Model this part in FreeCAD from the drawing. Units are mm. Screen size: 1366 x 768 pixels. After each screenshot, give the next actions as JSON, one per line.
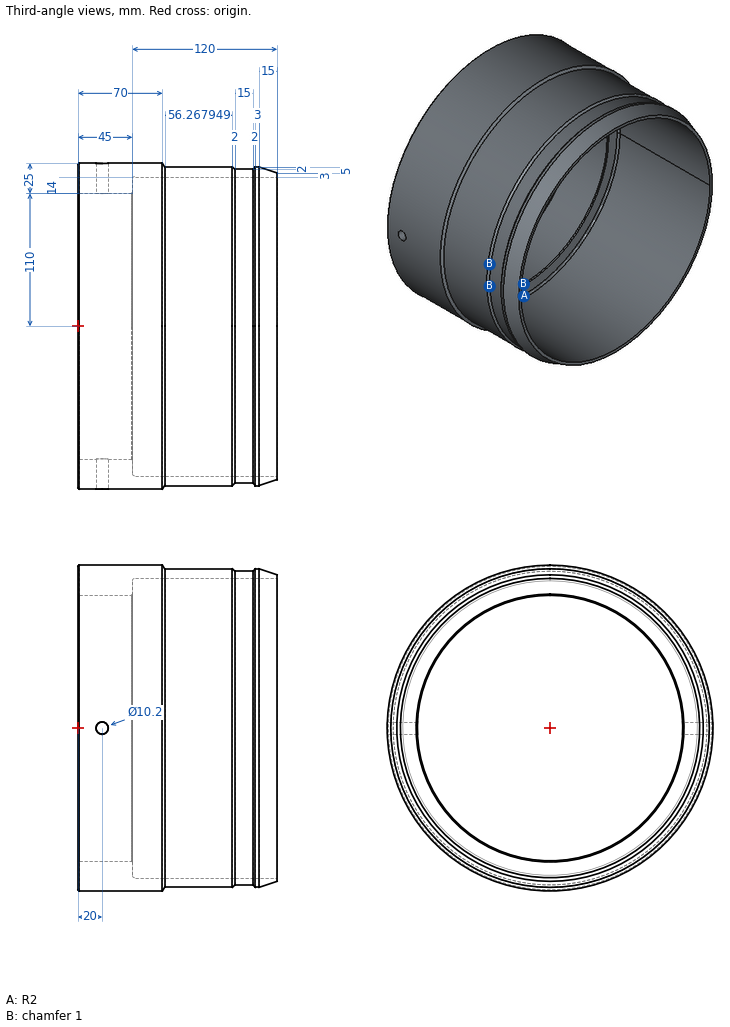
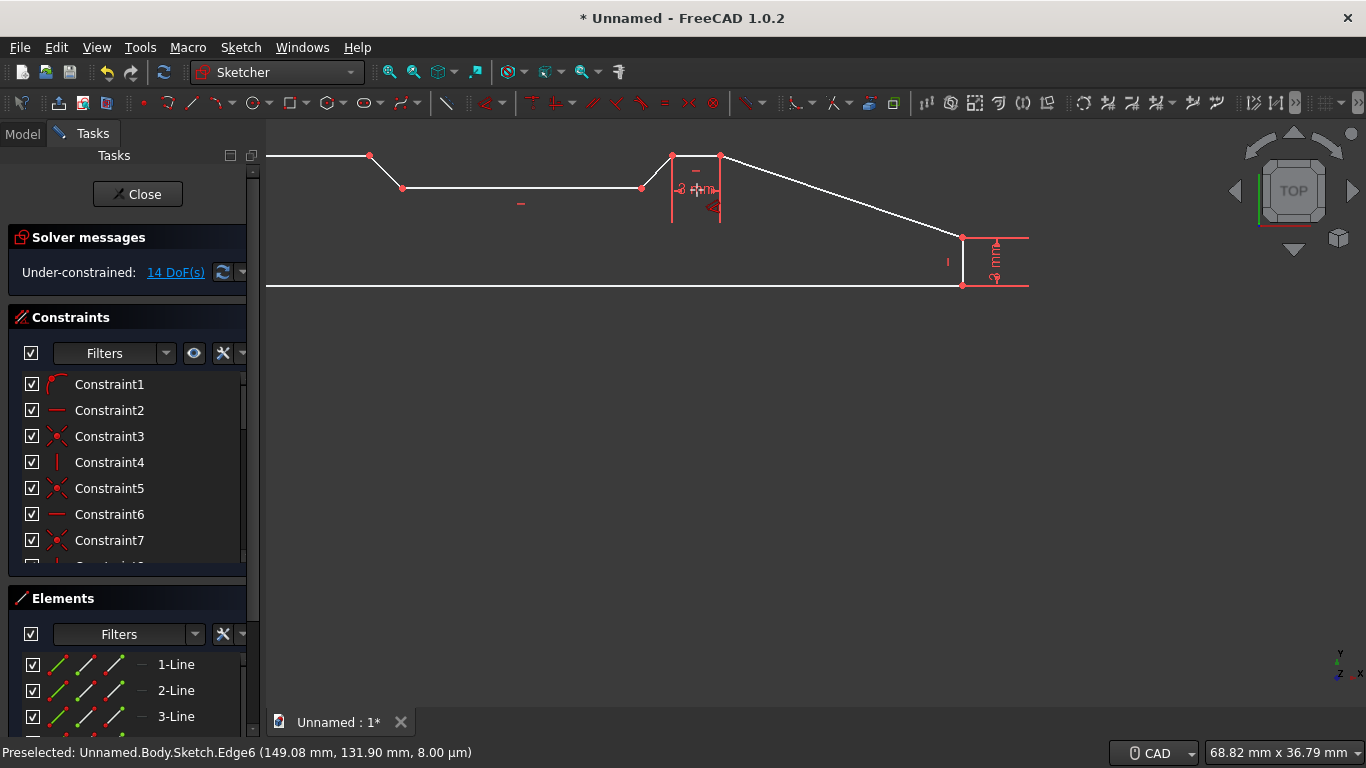
{"action": "scroll", "coordinate": [966, 260], "scroll_direction": "down", "scroll_amount": 9}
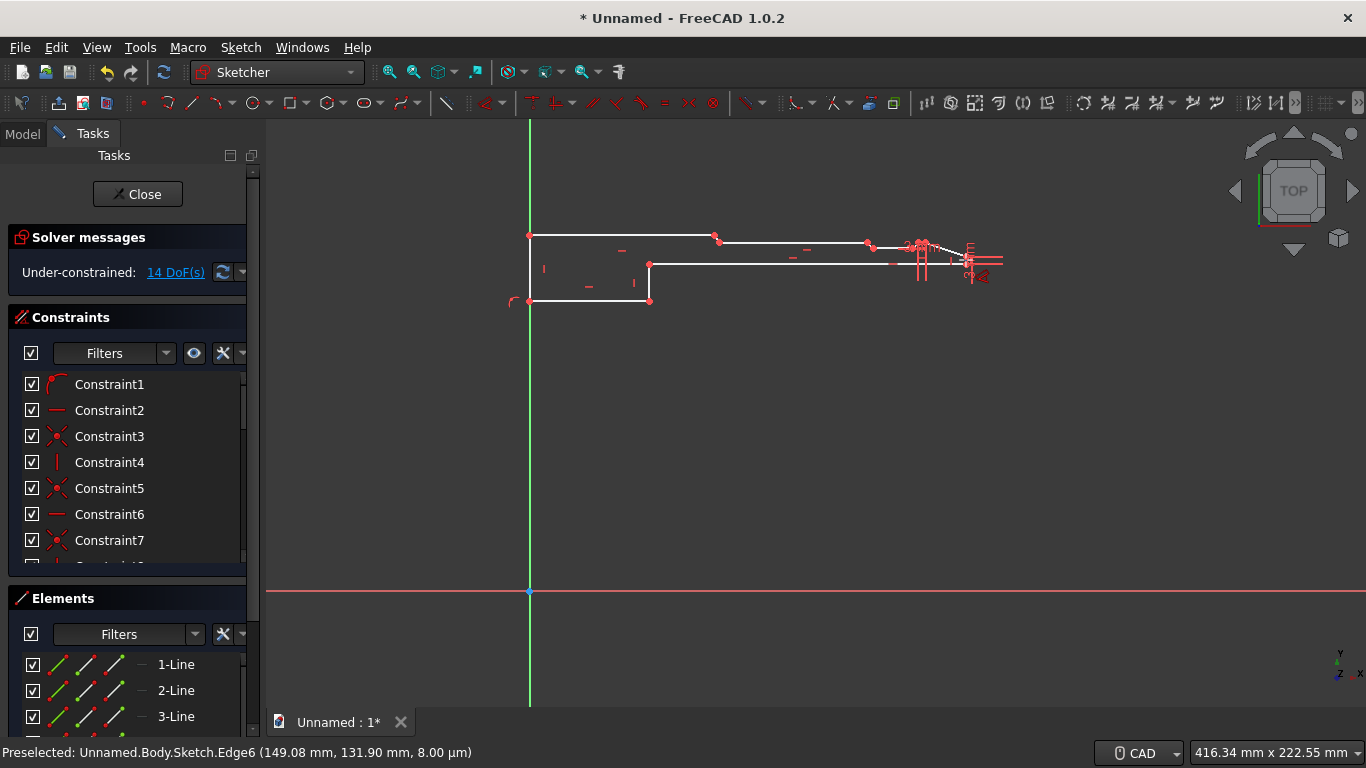
{"action": "left_click", "coordinate": [565, 301]}
{"action": "left_click", "coordinate": [589, 267]}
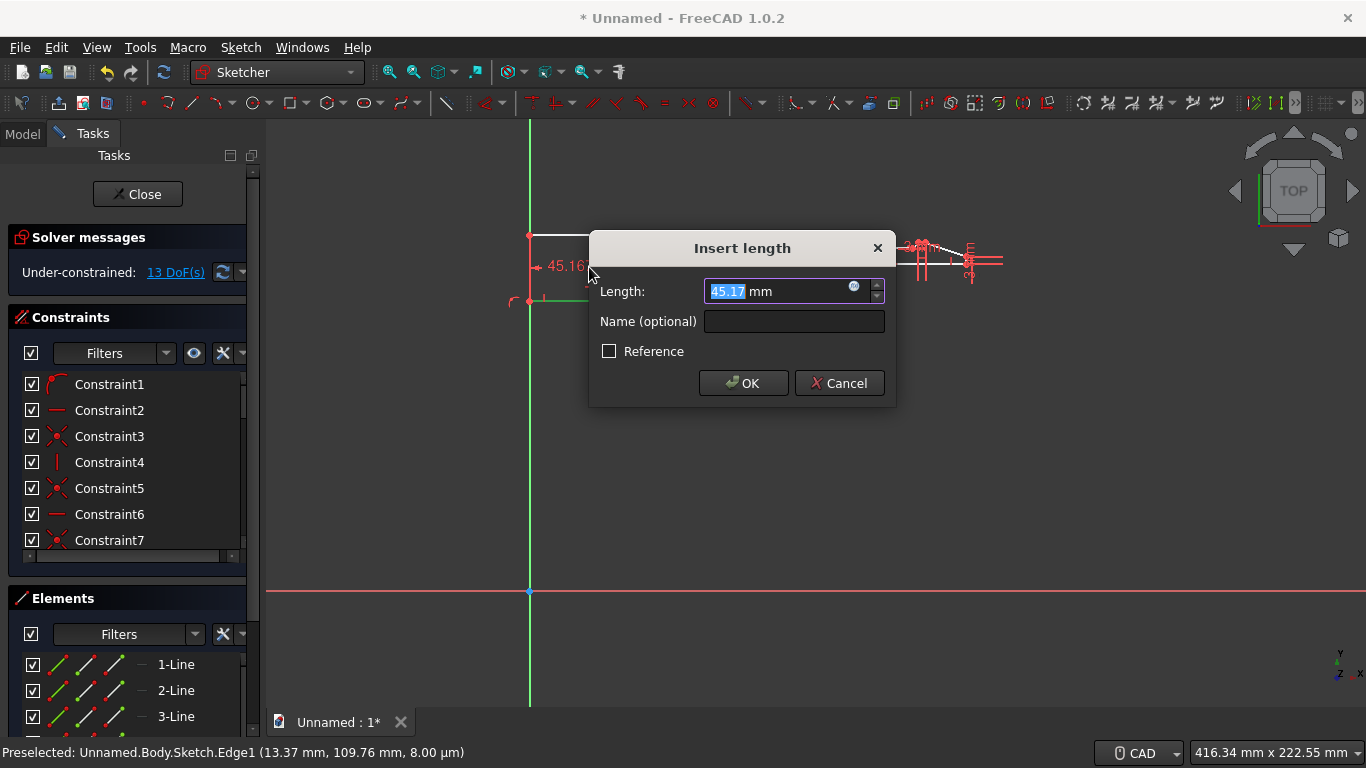
{"action": "type", "text": "45"}
{"action": "key", "text": "Return"}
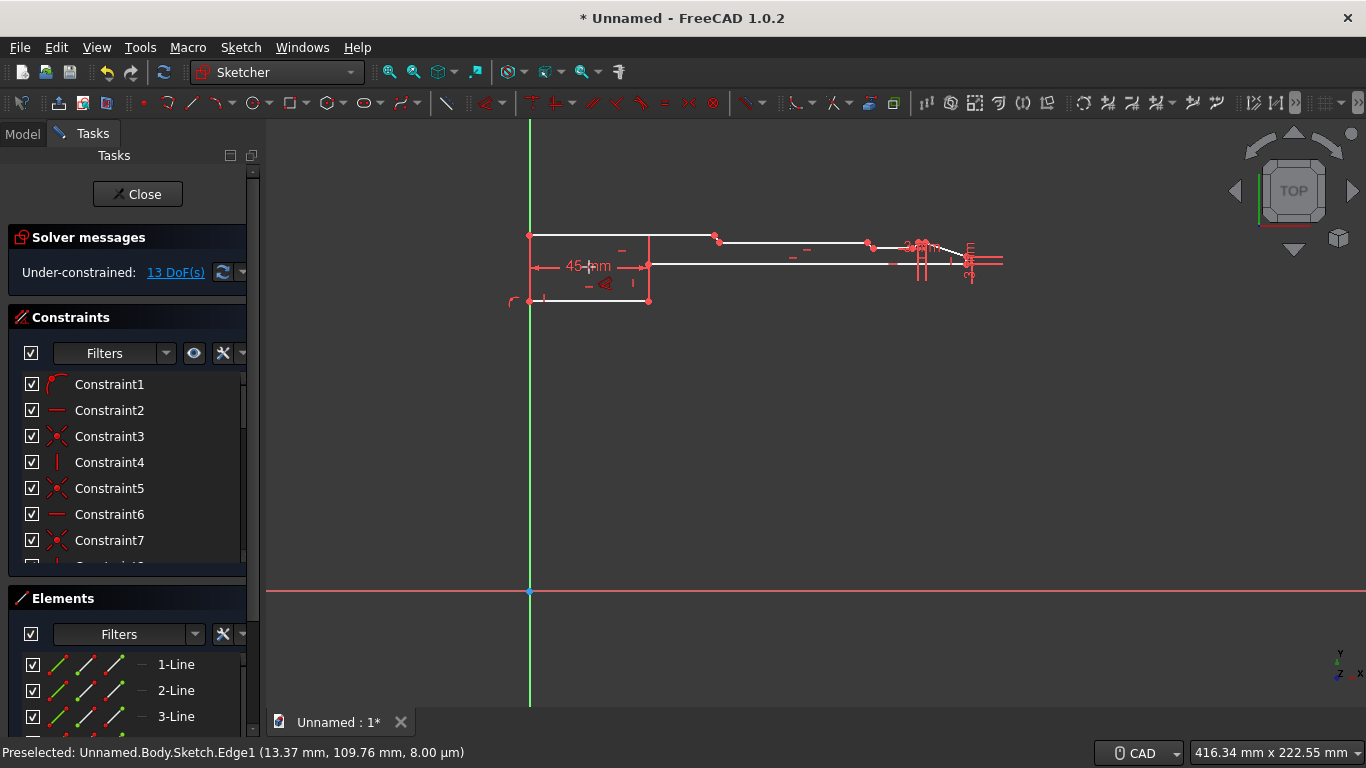
{"action": "scroll", "coordinate": [649, 290], "scroll_direction": "up", "scroll_amount": 2}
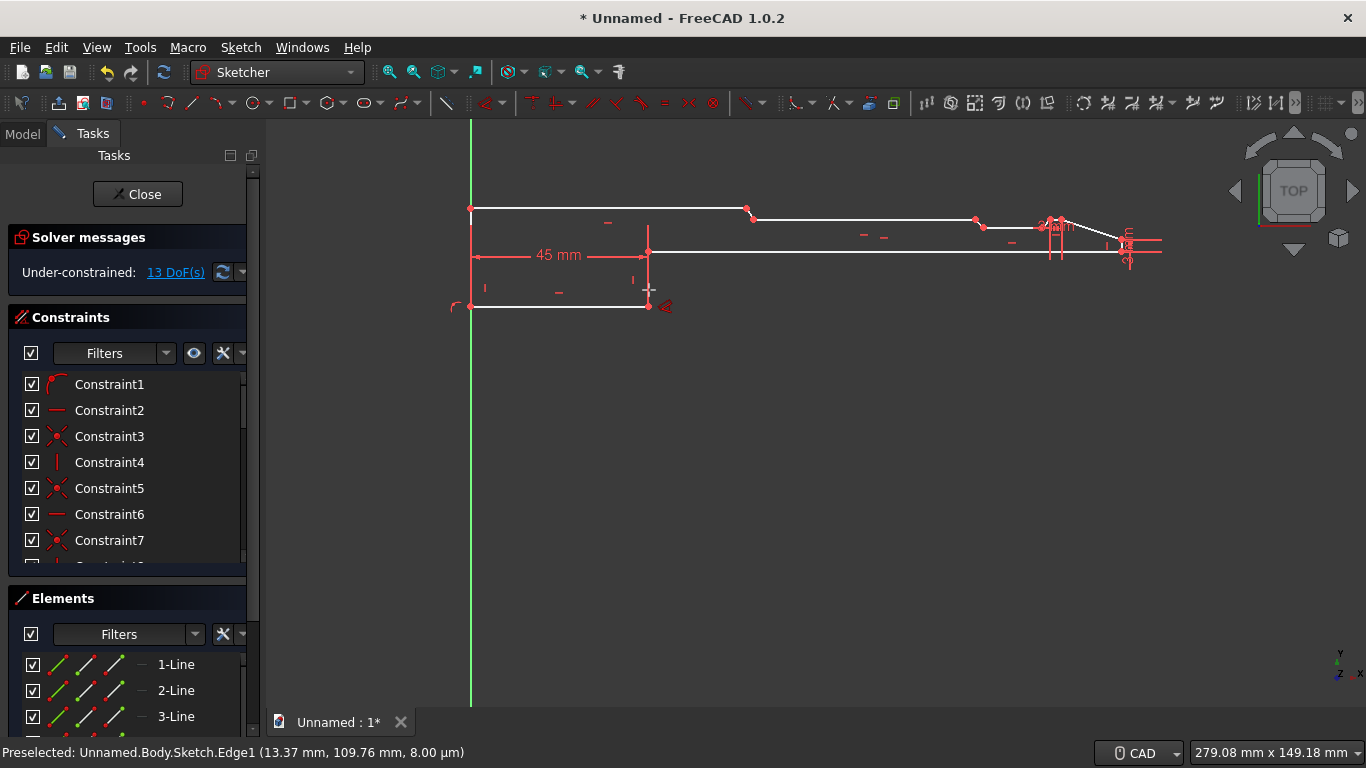
{"action": "left_click", "coordinate": [648, 290]}
{"action": "left_click", "coordinate": [614, 279]}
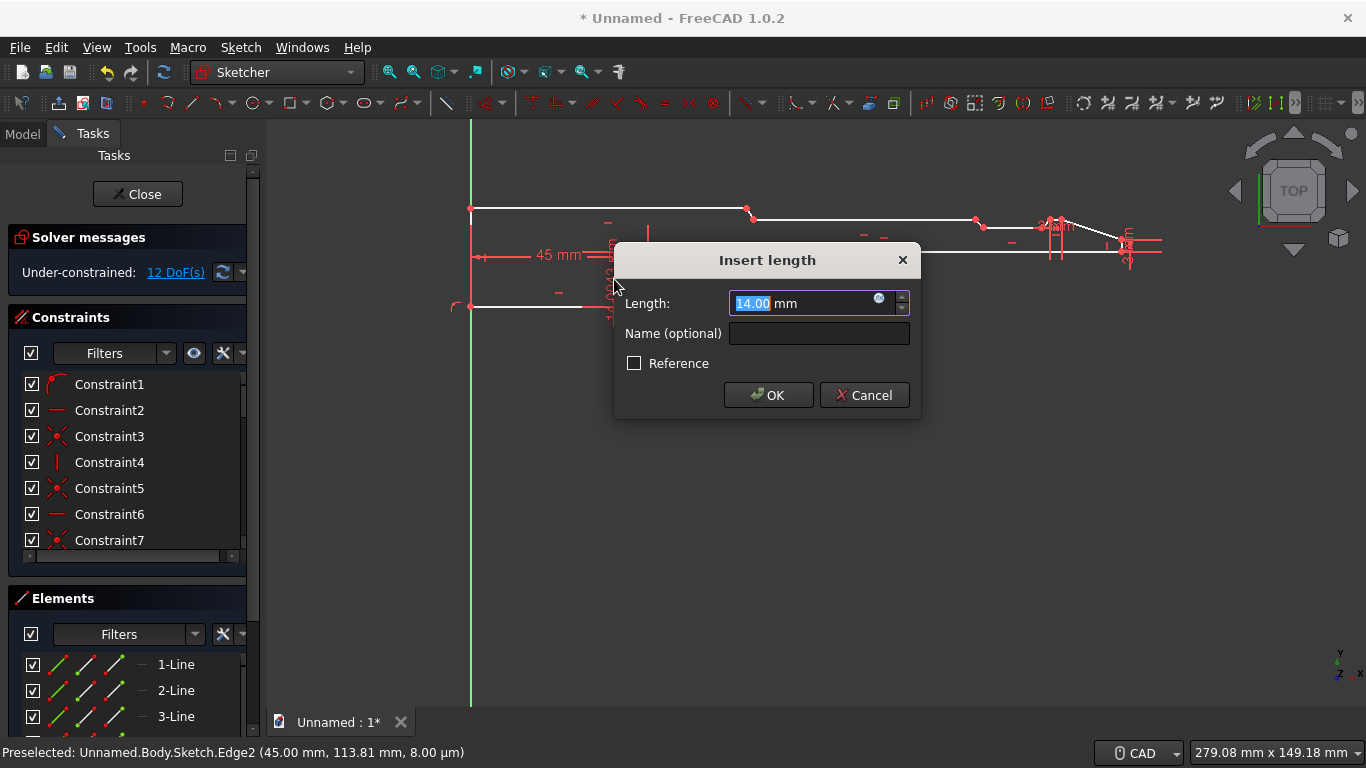
{"action": "type", "text": "14"}
{"action": "key", "text": "Return"}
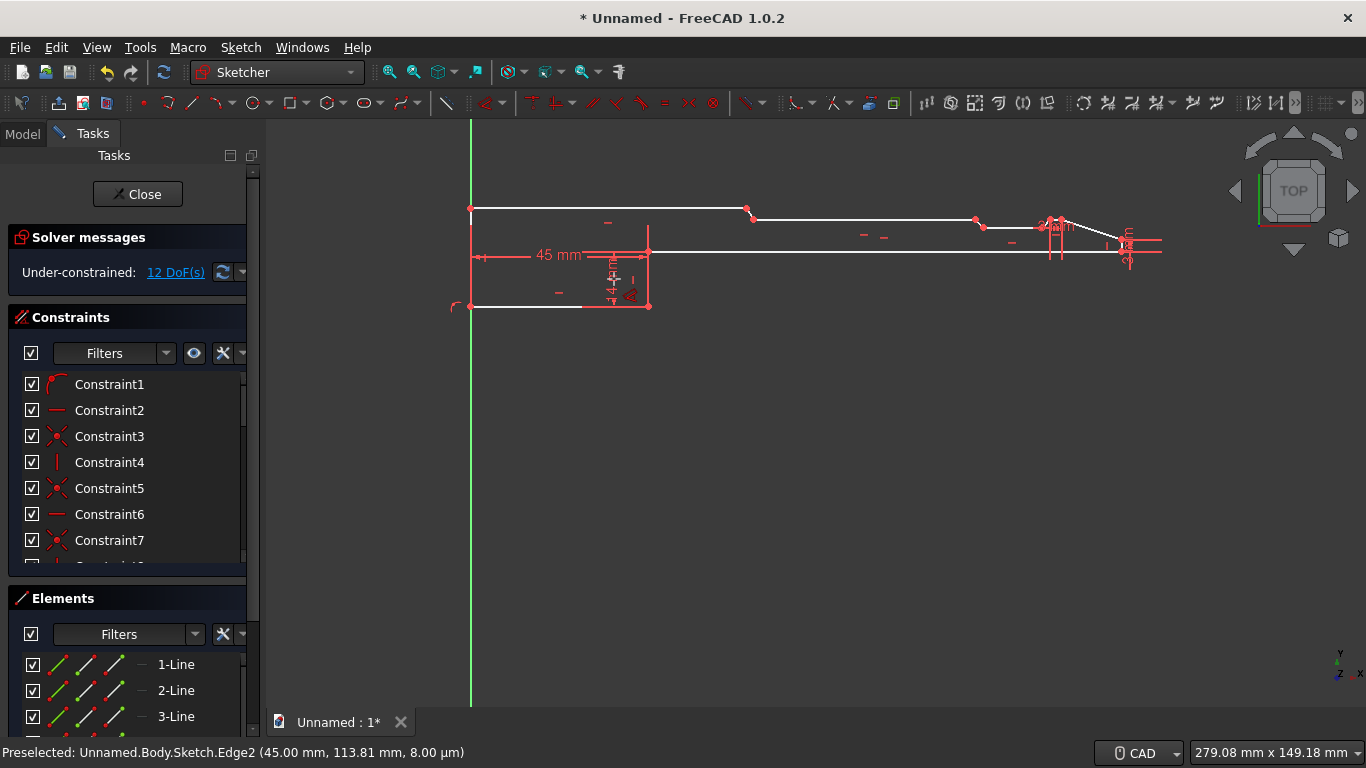
{"action": "left_click", "coordinate": [1025, 228]}
{"action": "left_click", "coordinate": [1013, 194]}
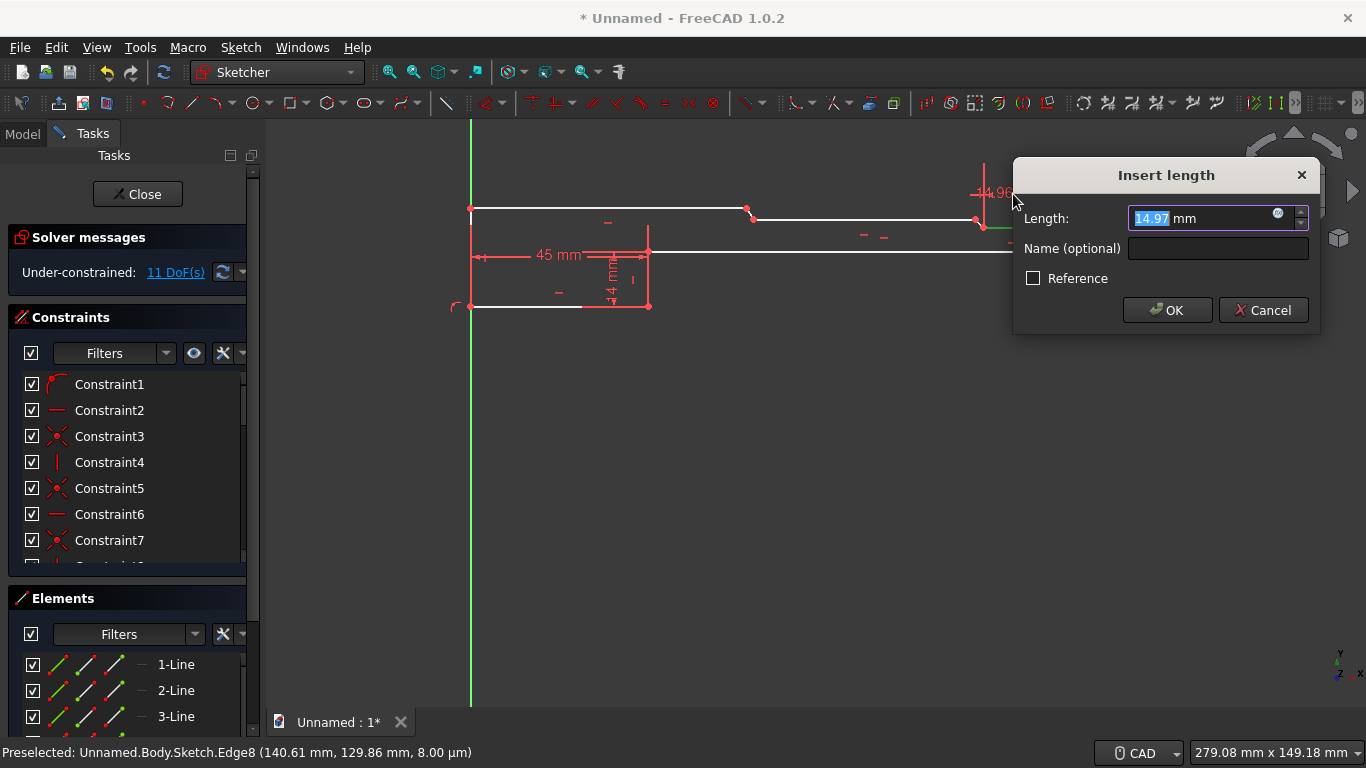
{"action": "type", "text": "15"}
{"action": "key", "text": "Return"}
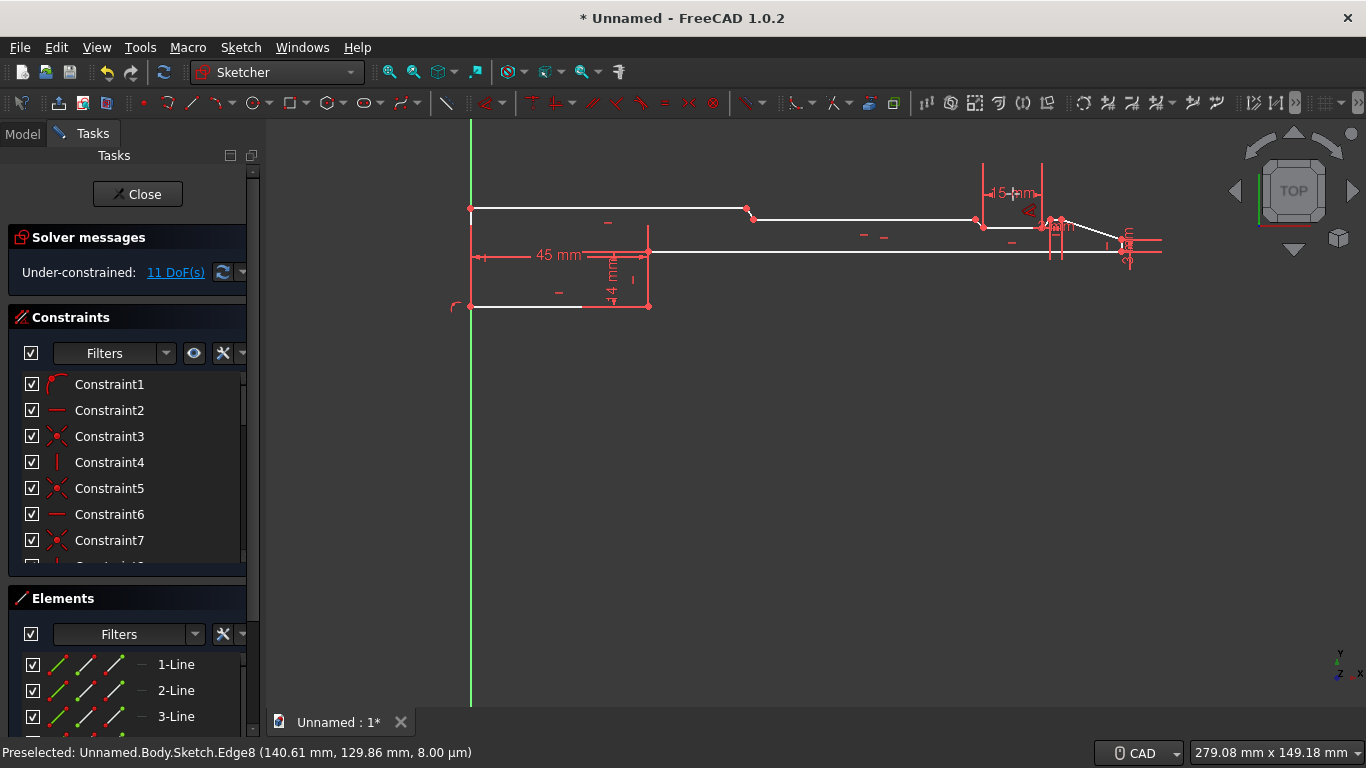
{"action": "left_click", "coordinate": [664, 208]}
{"action": "left_click", "coordinate": [609, 174]}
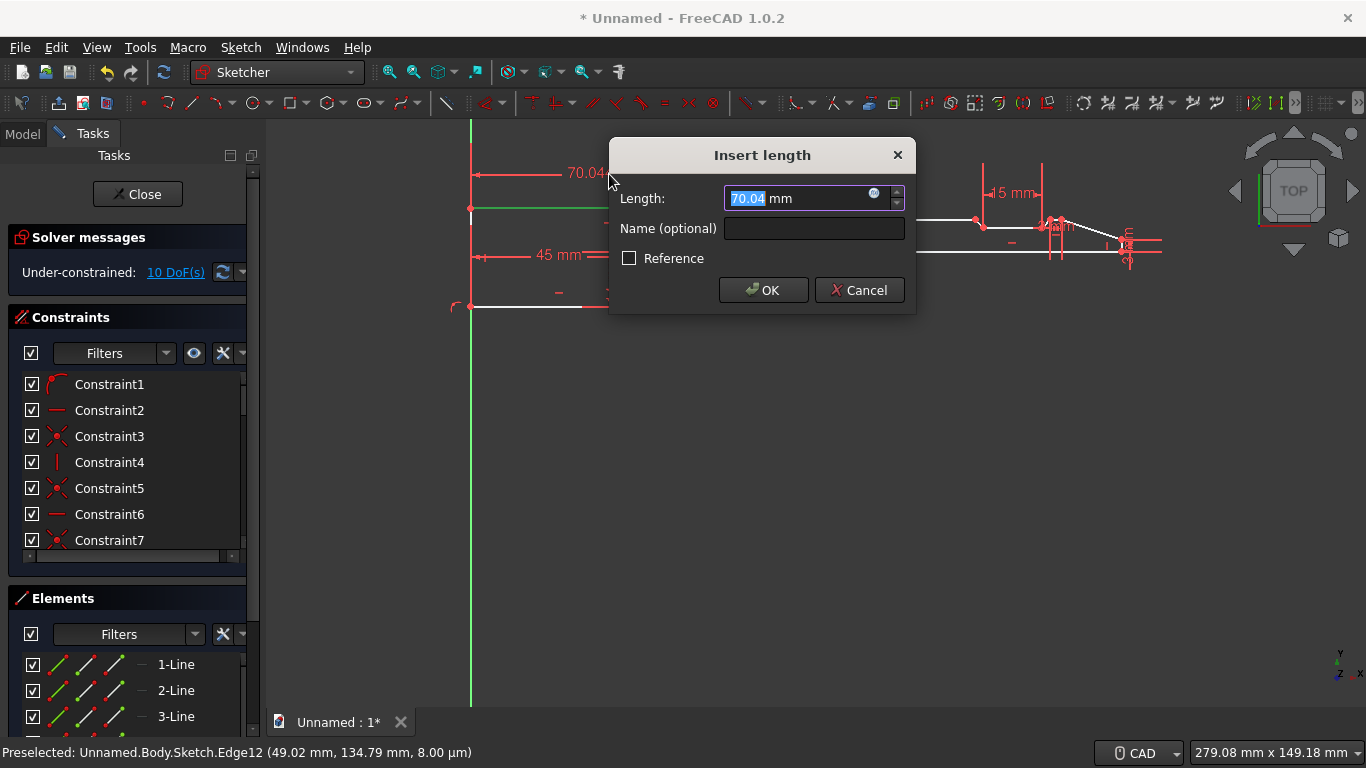
{"action": "type", "text": "70"}
{"action": "key", "text": "Return"}